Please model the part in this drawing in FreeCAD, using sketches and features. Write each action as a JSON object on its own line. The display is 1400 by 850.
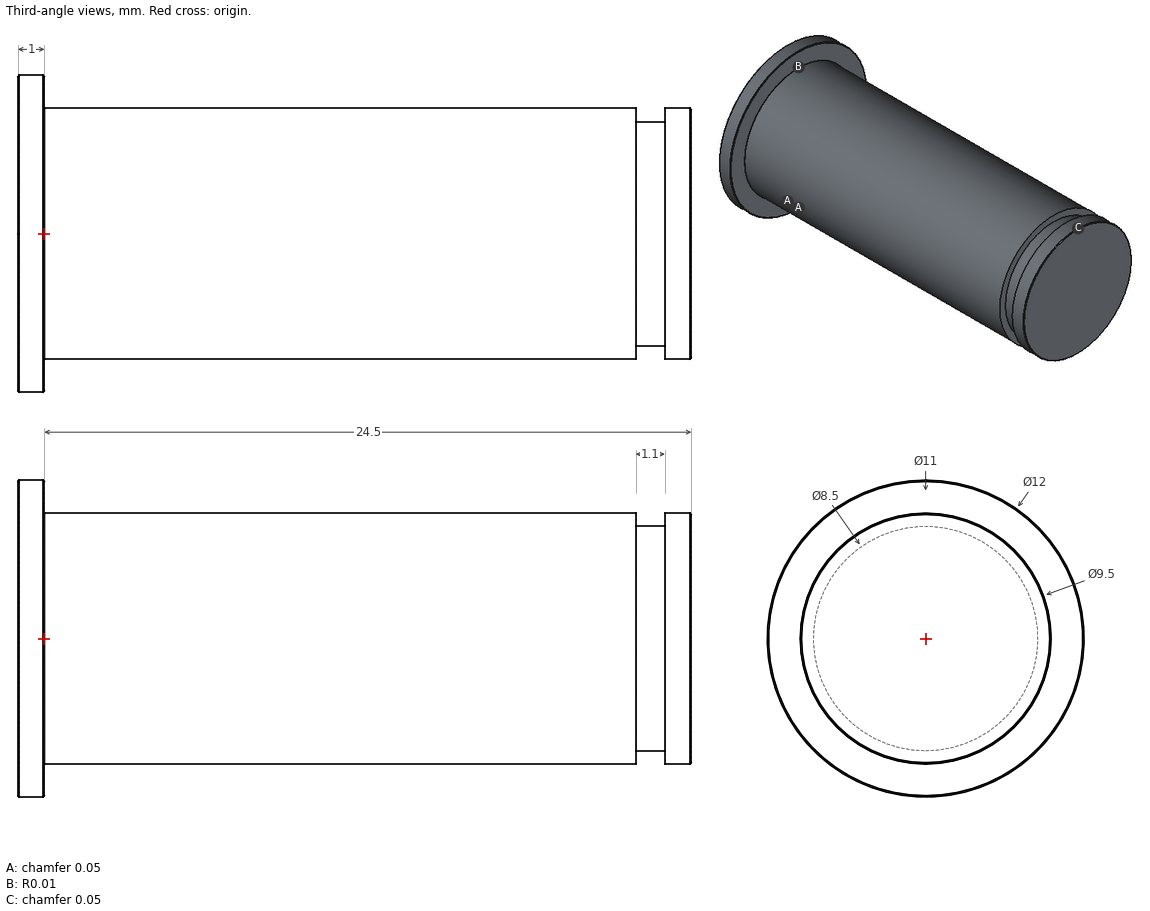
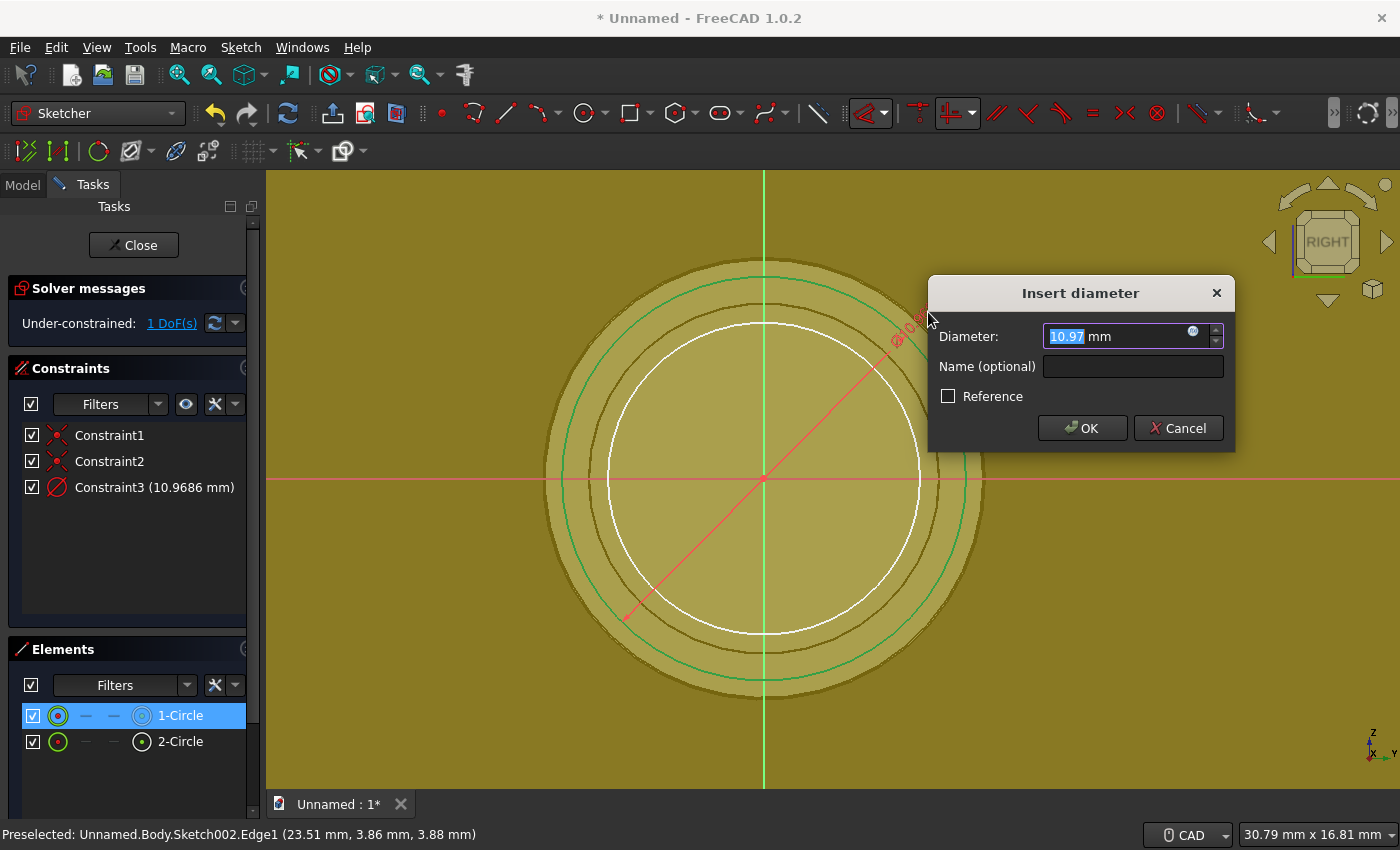
{"action": "type", "text": "11"}
{"action": "key", "text": "Return"}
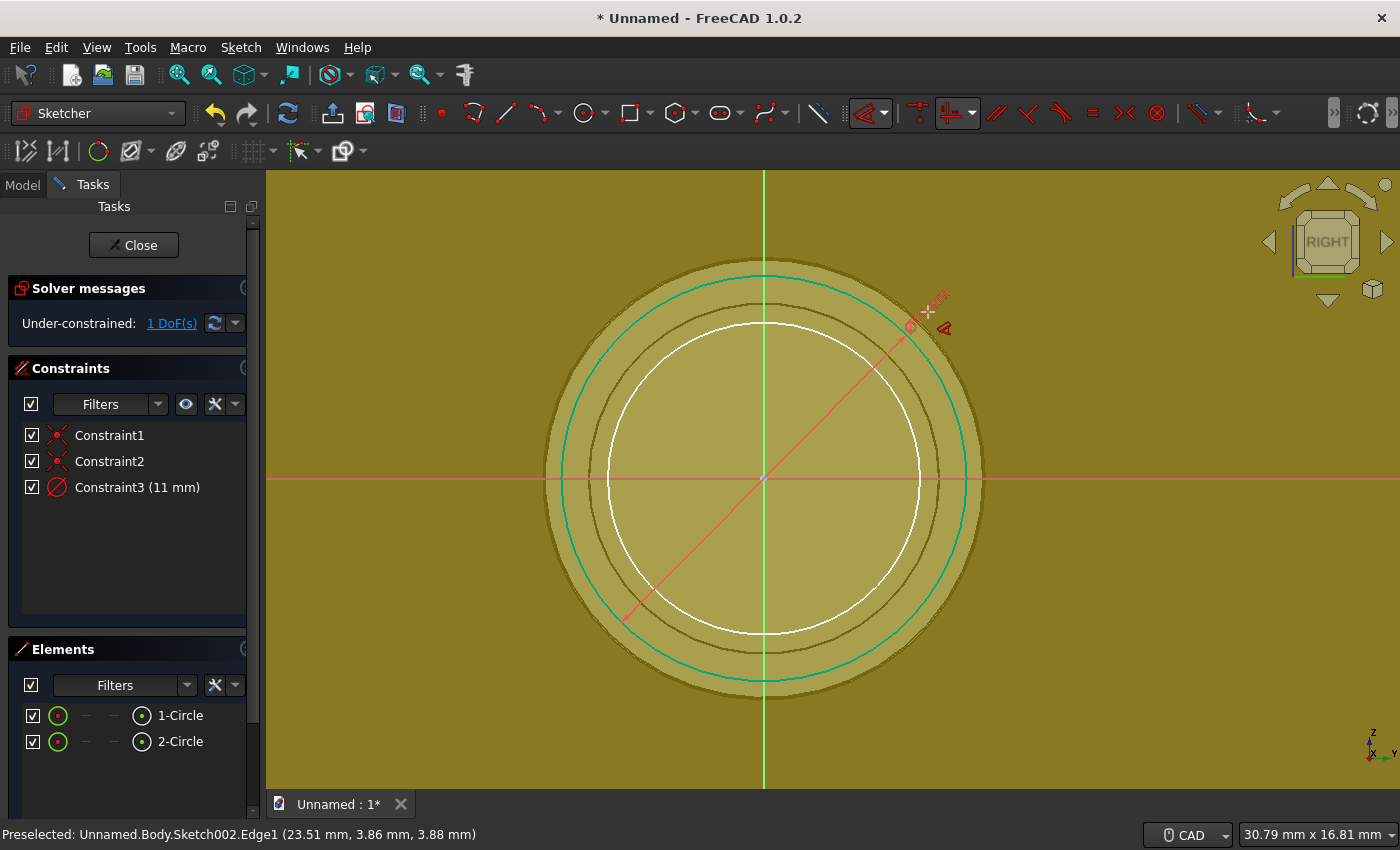
{"action": "left_click", "coordinate": [874, 368]}
{"action": "left_click", "coordinate": [897, 345]}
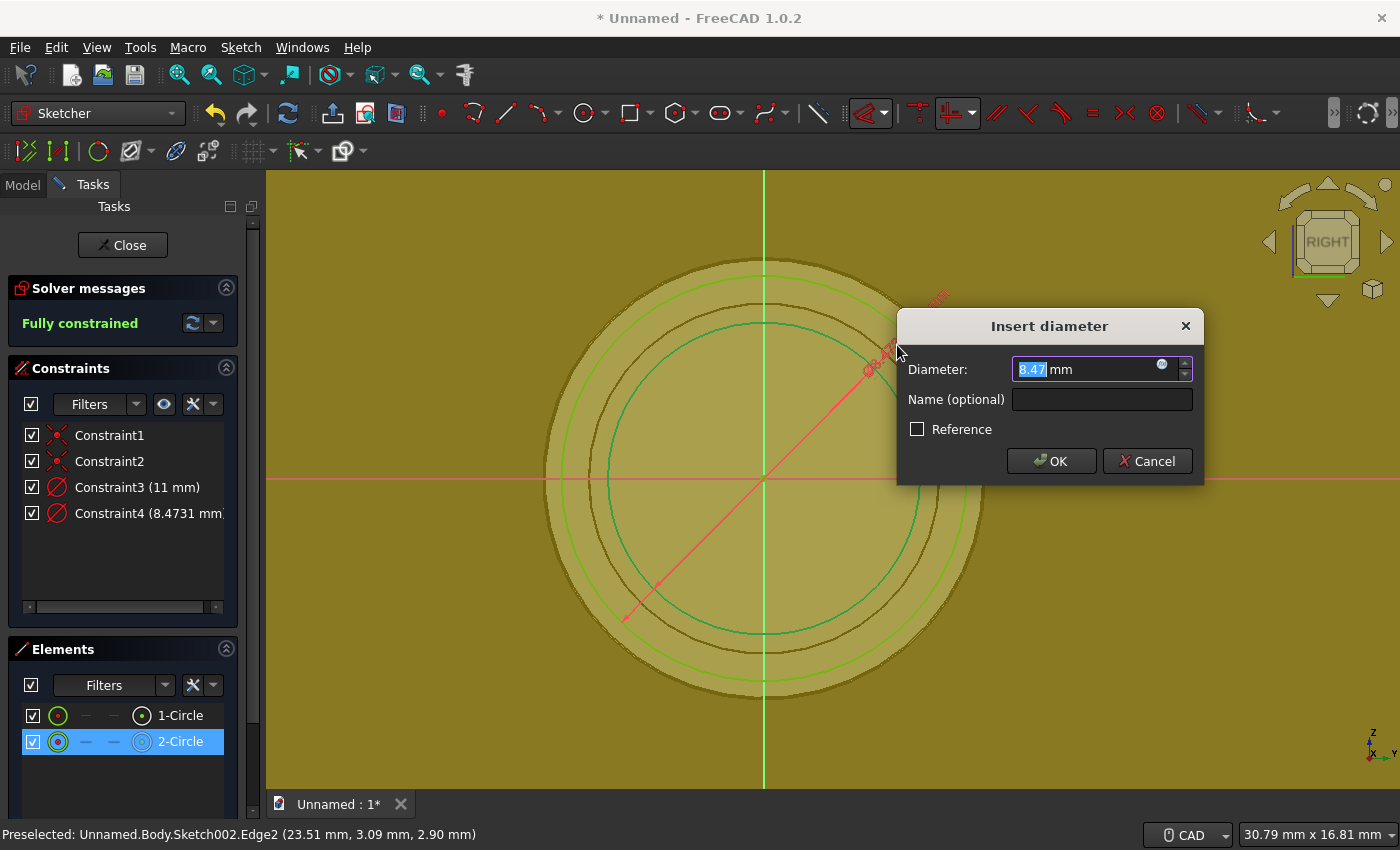
{"action": "type", "text": "8.5"}
{"action": "key", "text": "Return"}
{"action": "key", "text": "Escape"}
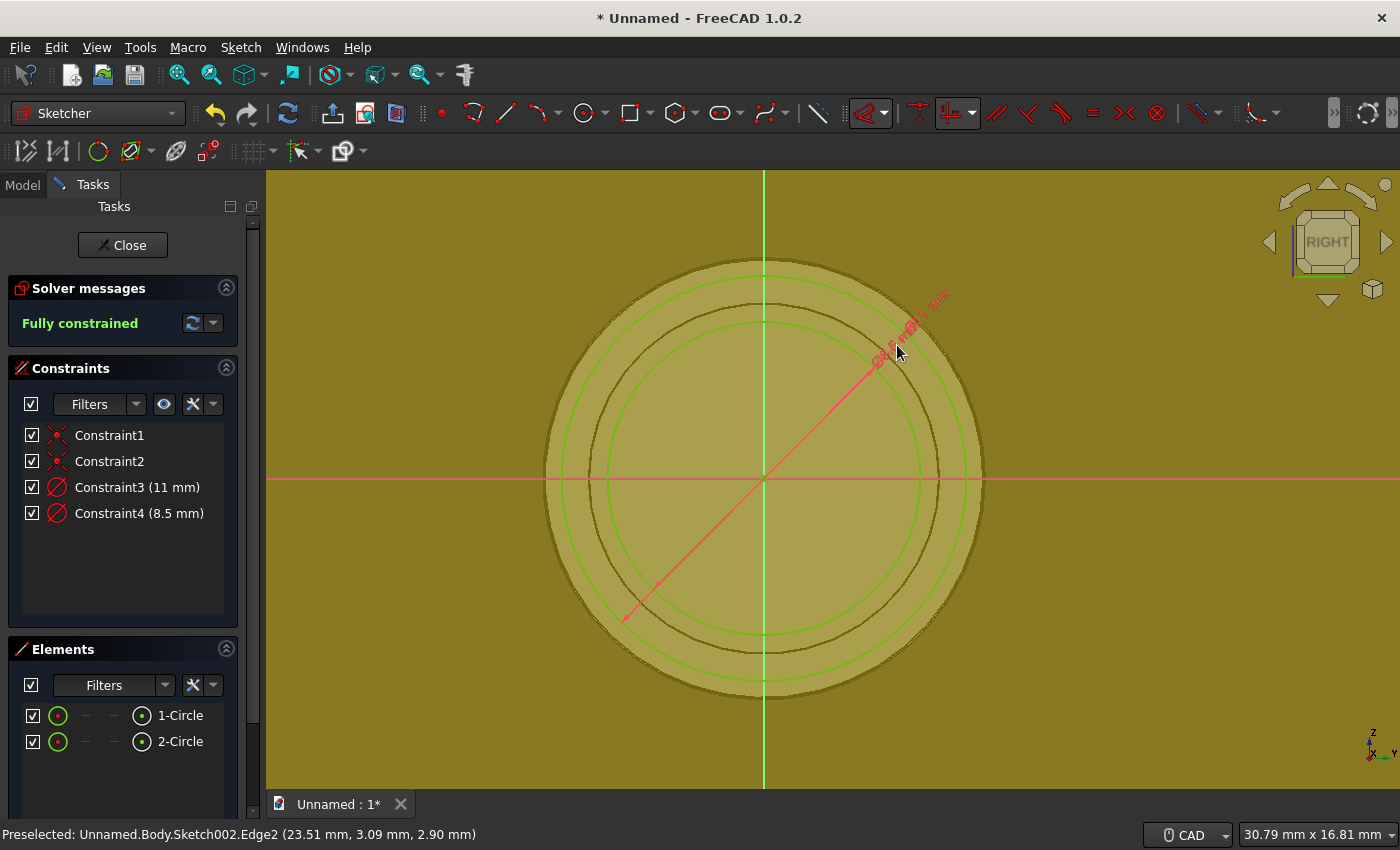
{"action": "left_click", "coordinate": [123, 245]}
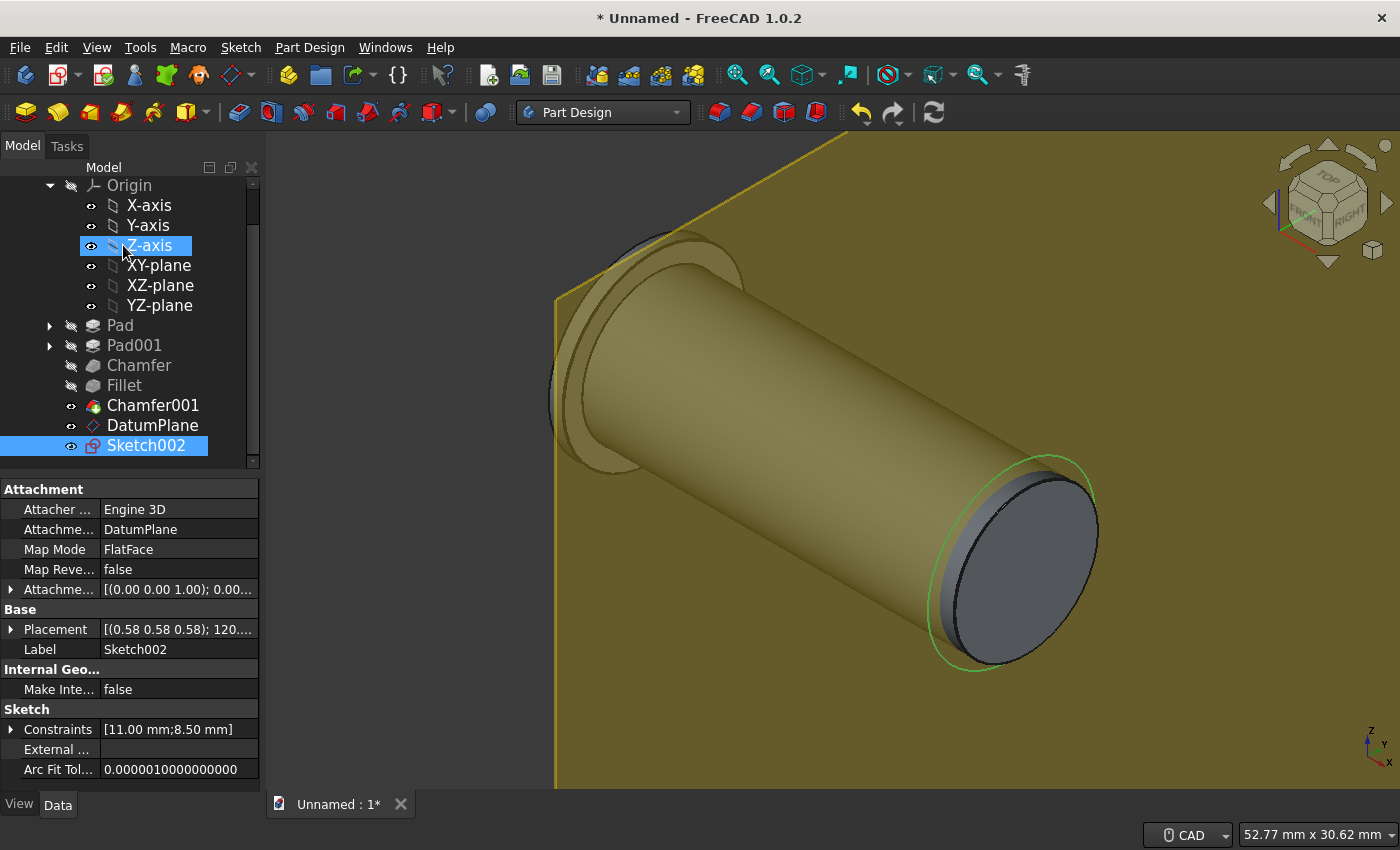
{"action": "left_click", "coordinate": [240, 112]}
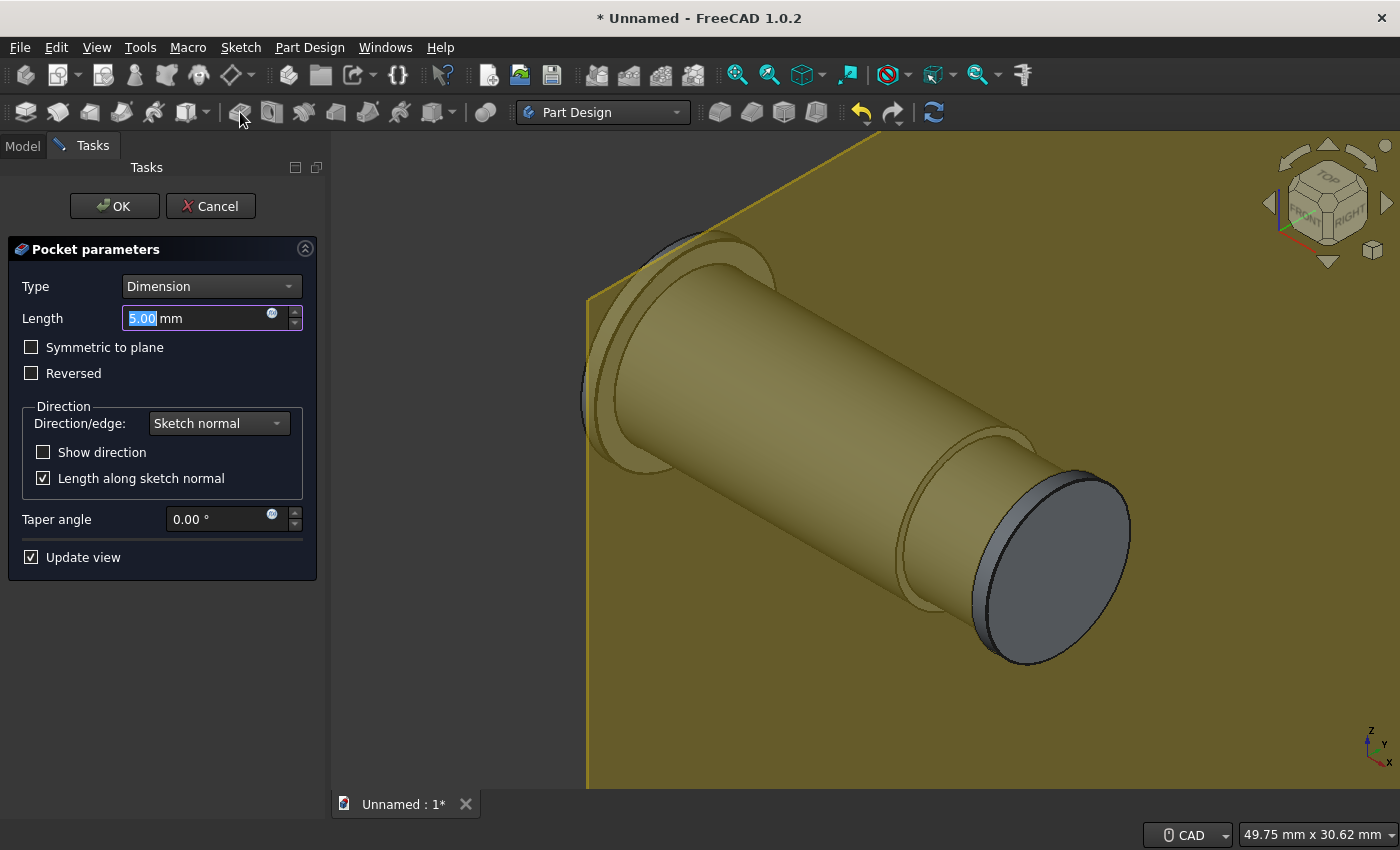
{"action": "type", "text": "1.1"}
{"action": "key", "text": "Tab"}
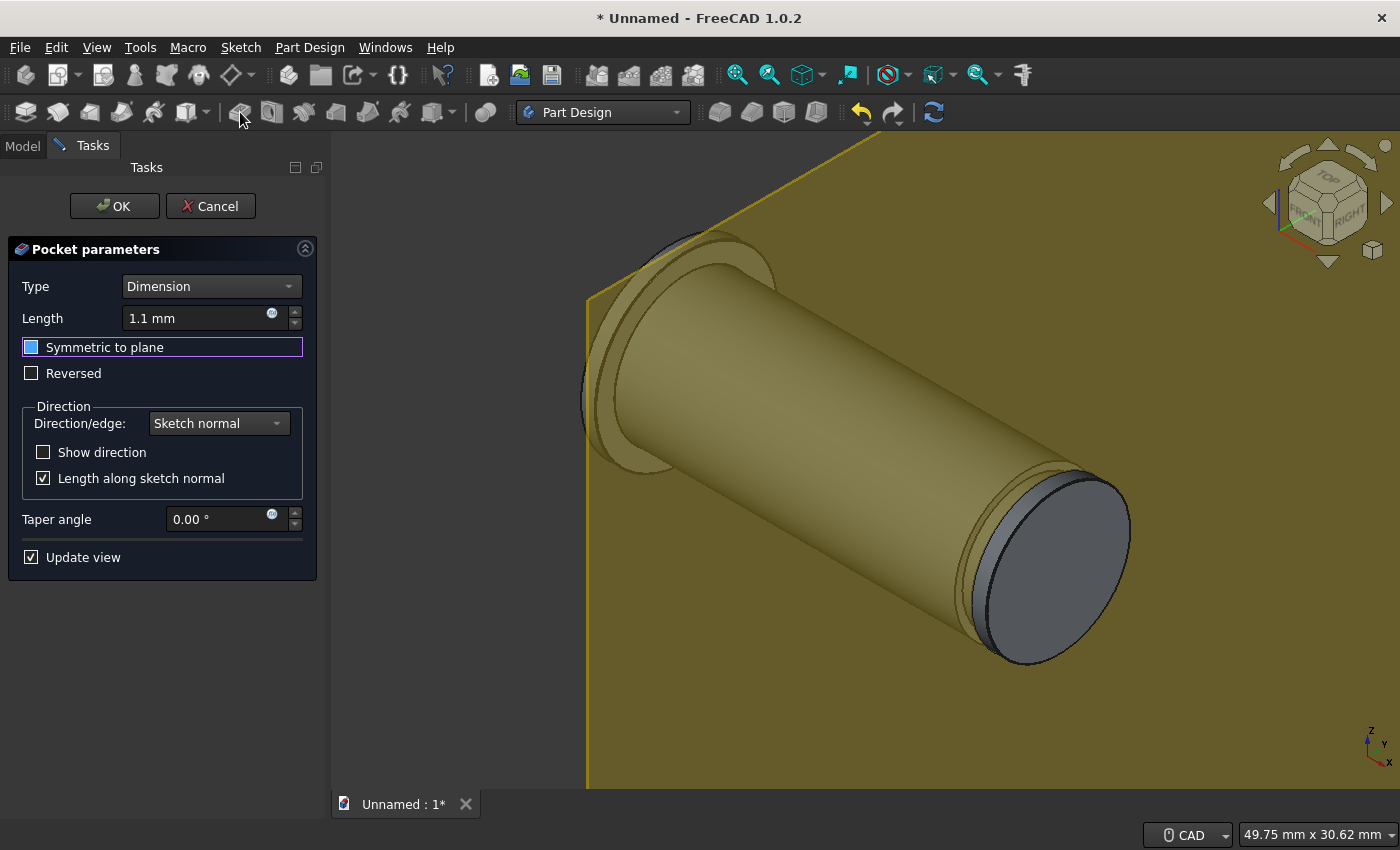
{"action": "left_click", "coordinate": [115, 206]}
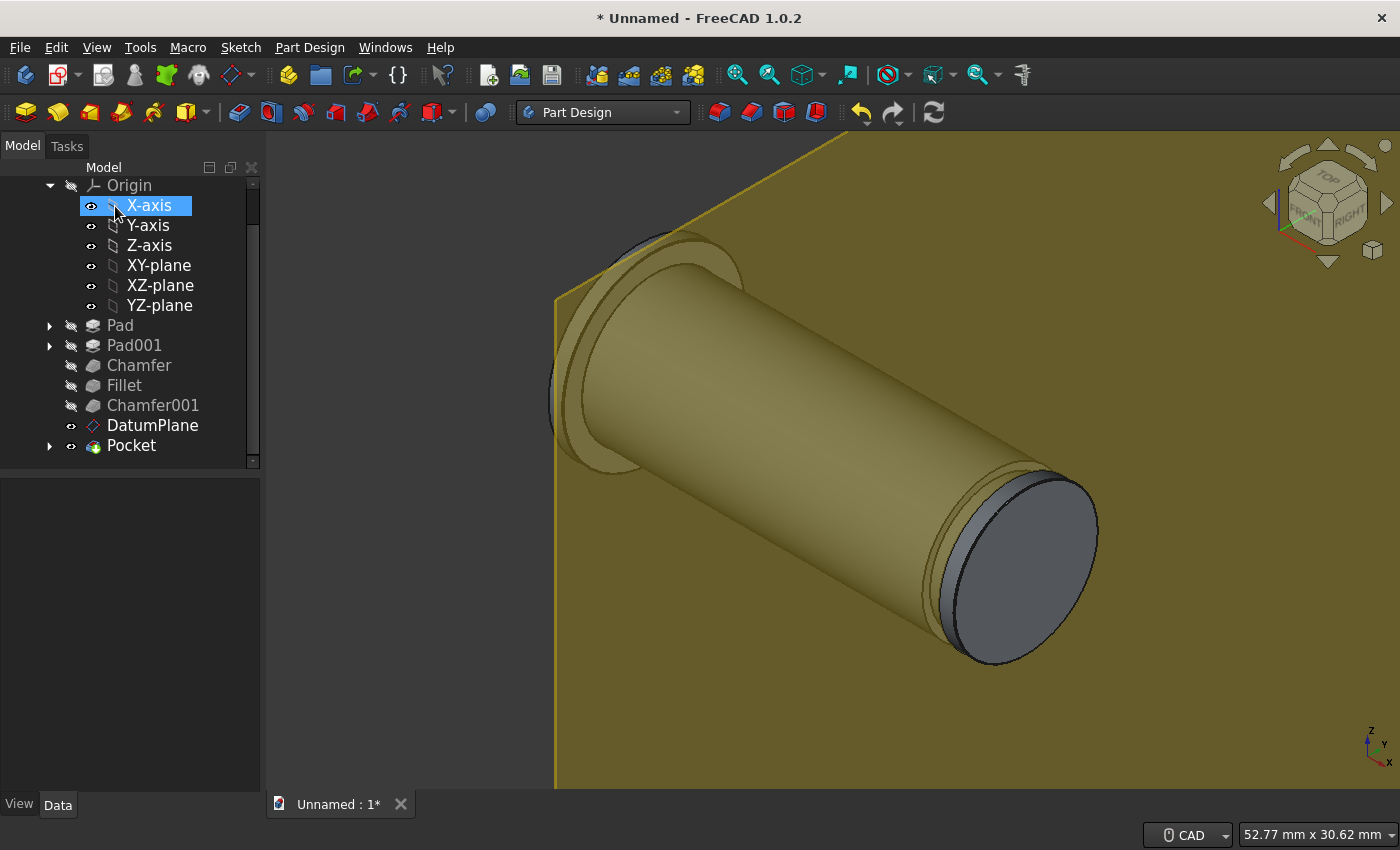
{"action": "left_click", "coordinate": [116, 426]}
{"action": "key", "text": "space"}